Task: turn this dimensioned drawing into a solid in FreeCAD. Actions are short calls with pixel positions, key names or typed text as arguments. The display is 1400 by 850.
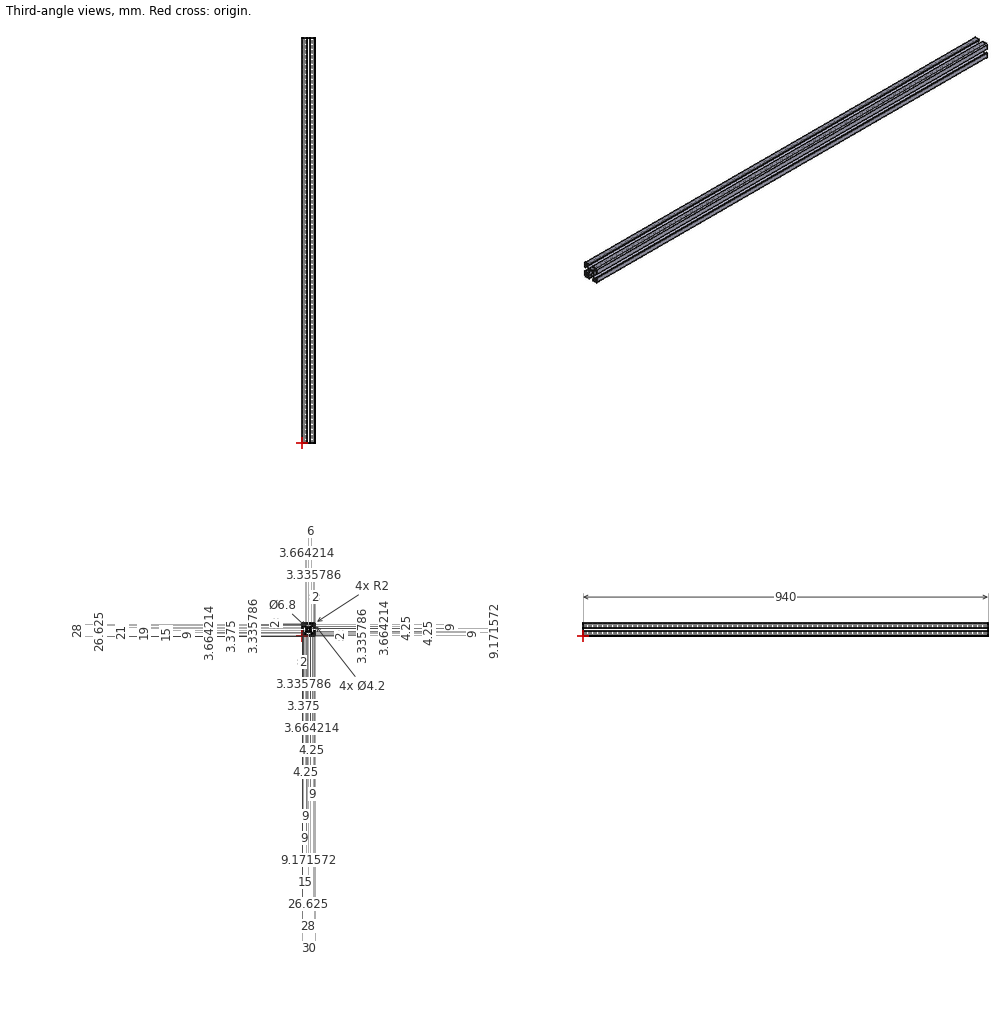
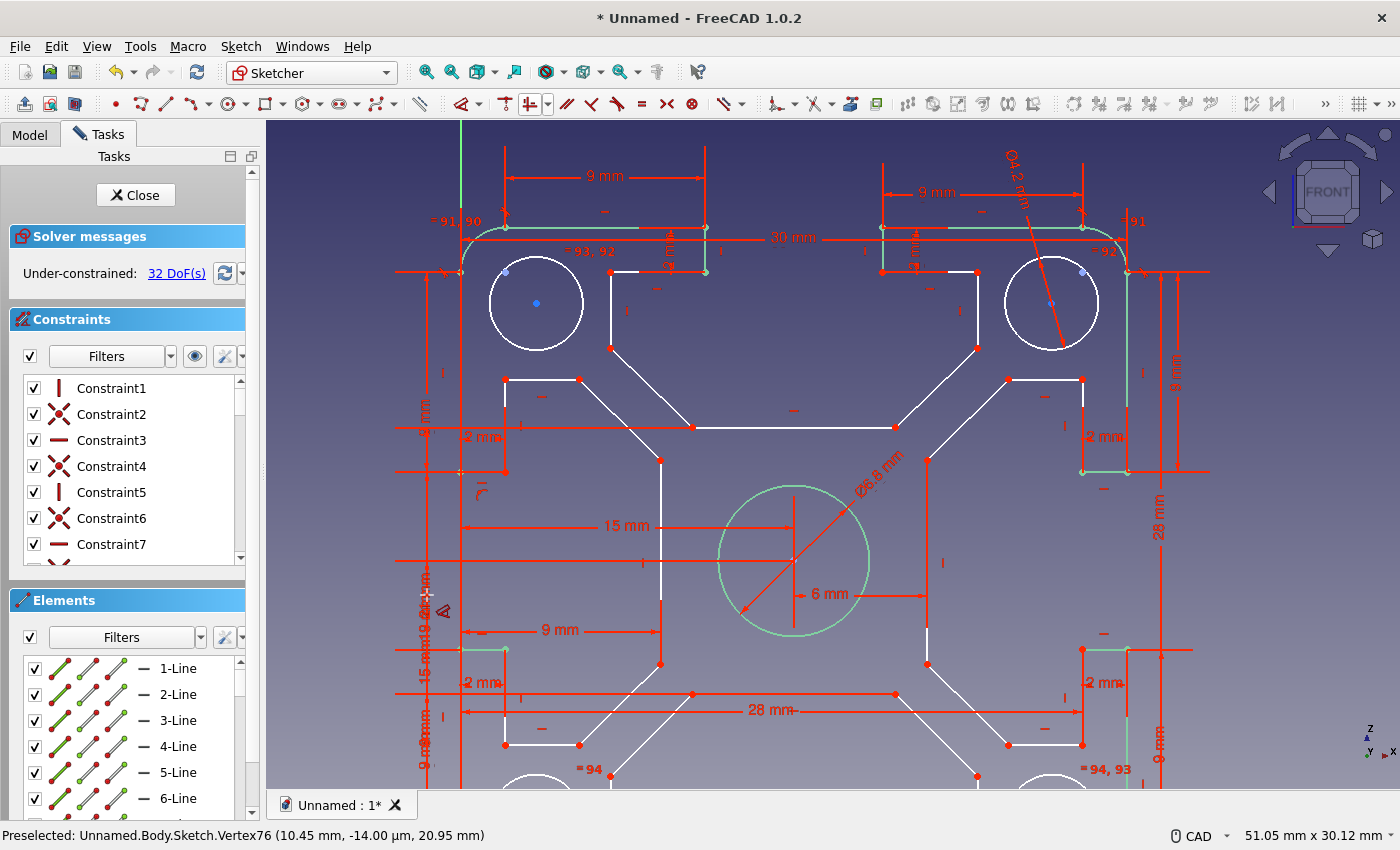
click(1083, 444)
click(1049, 405)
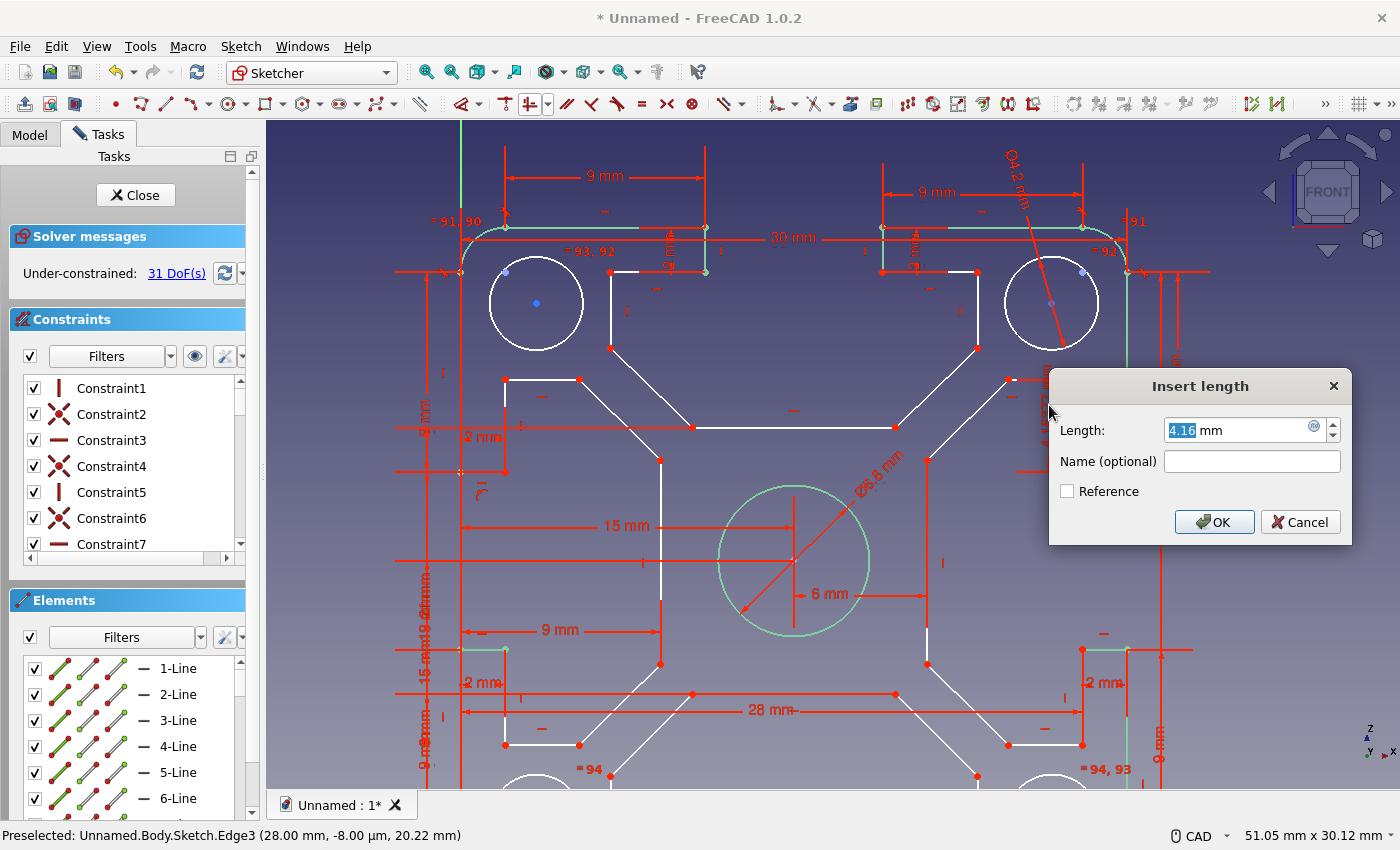
text(4.25)
key(Return)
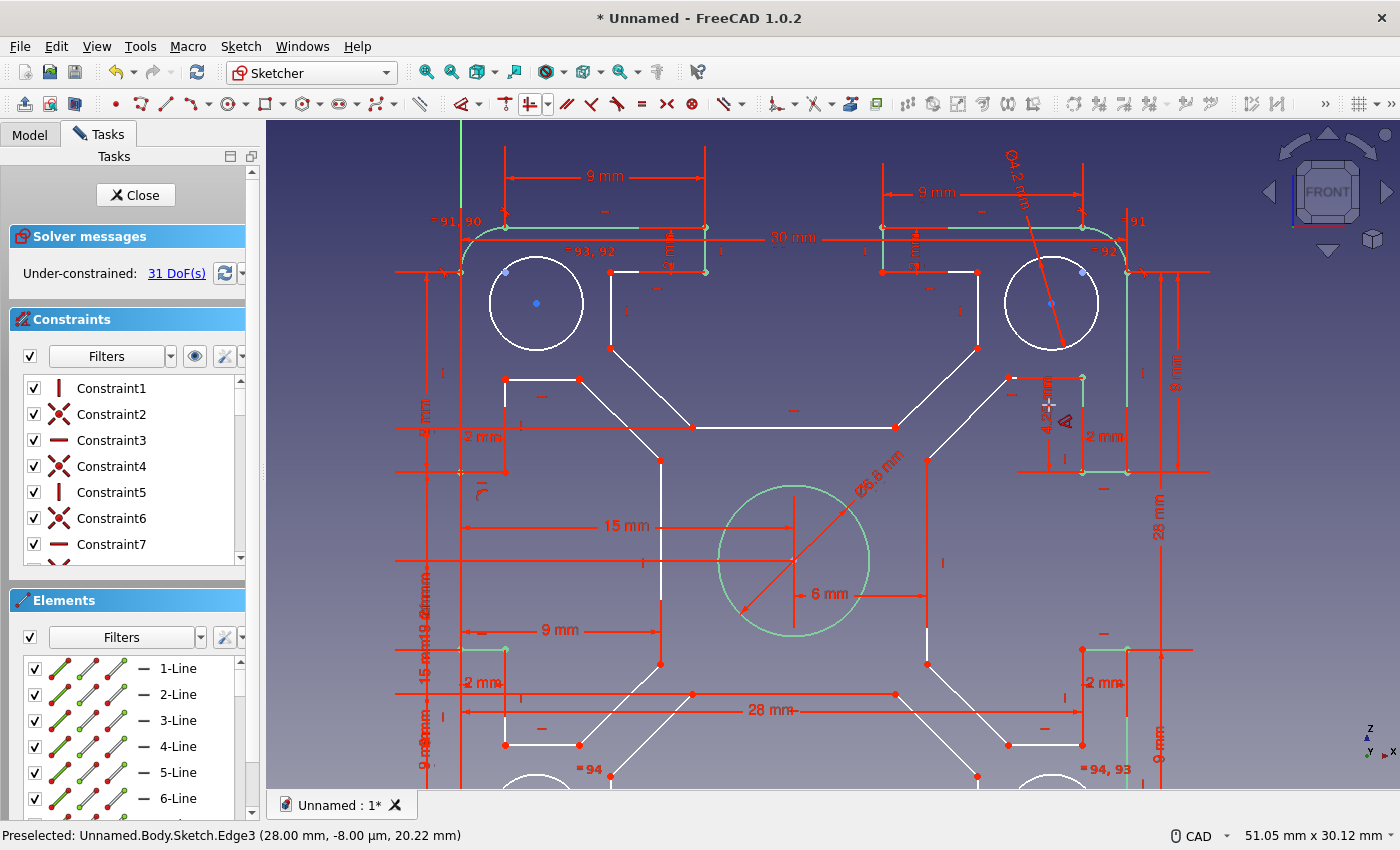
click(1083, 717)
click(1049, 719)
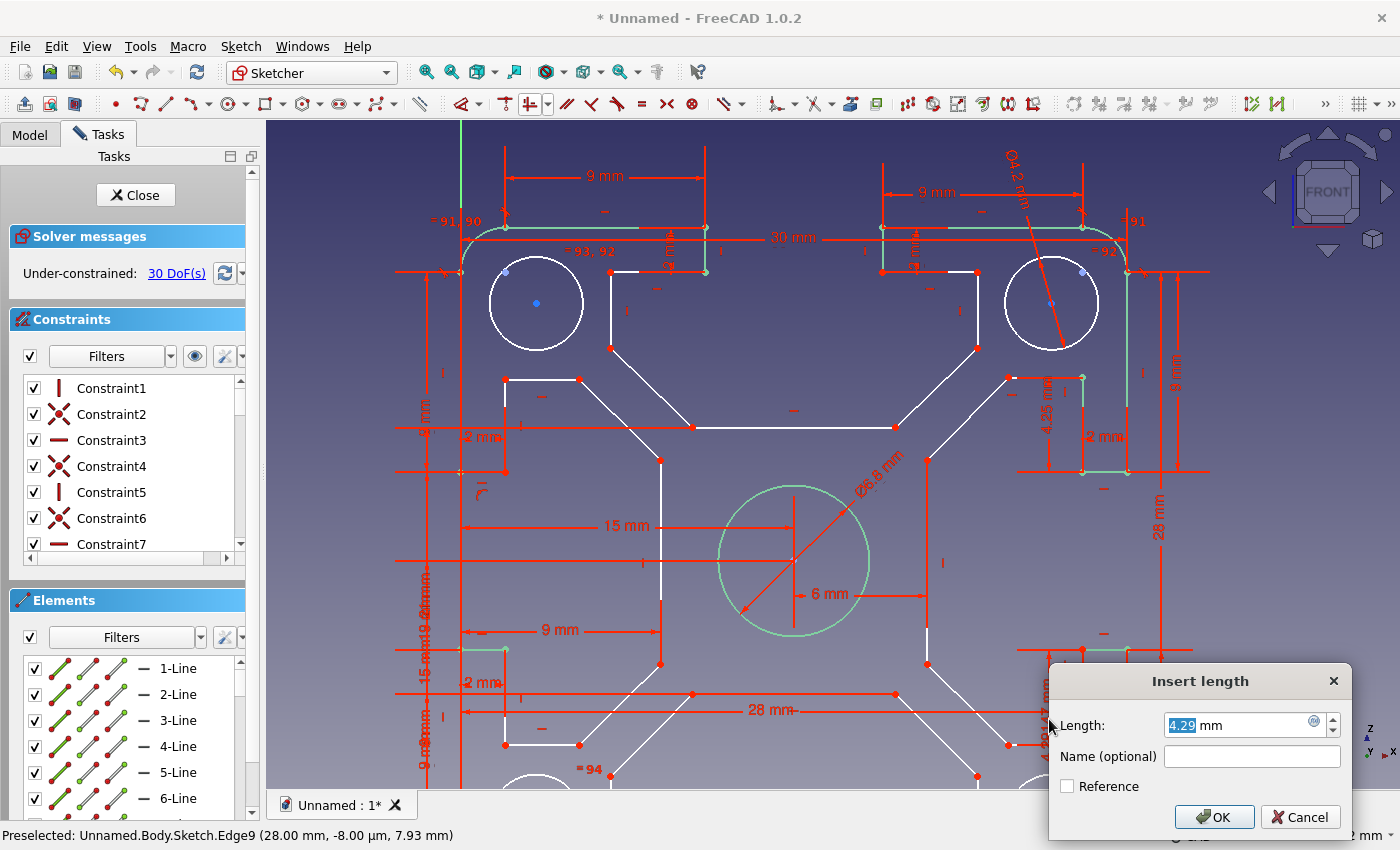
text(4.25)
key(Return)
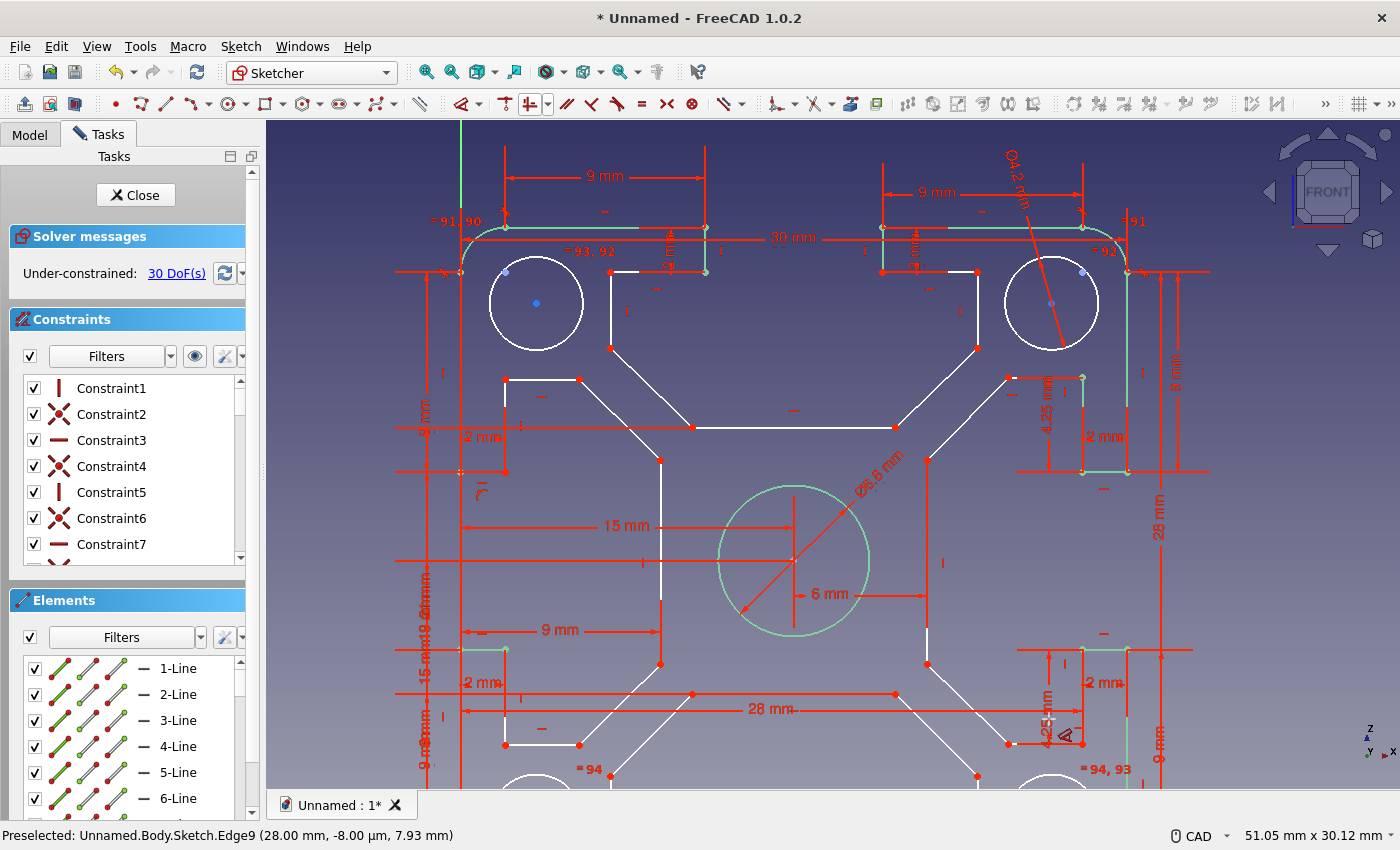
scroll(705, 238, down, 2)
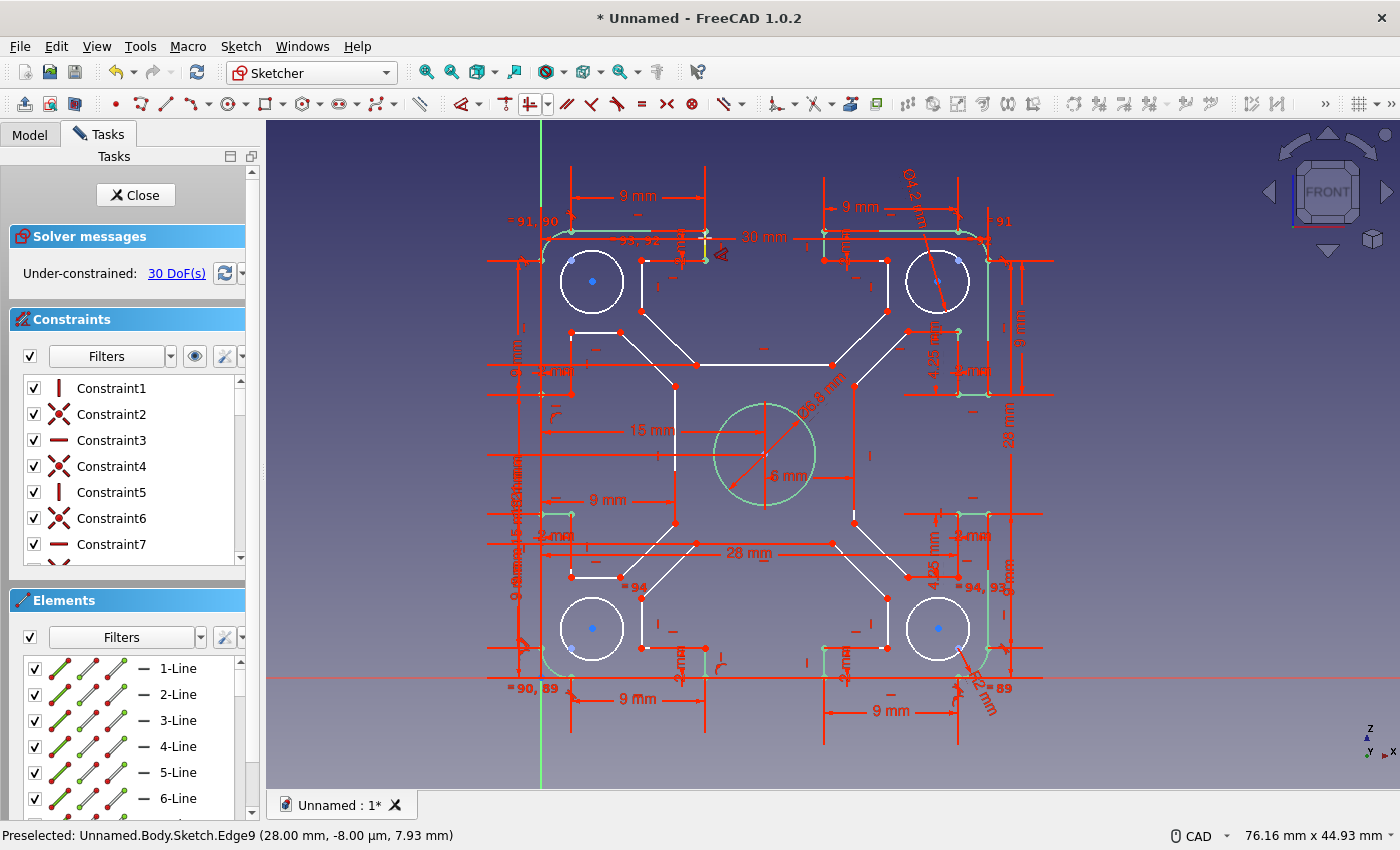
click(843, 648)
click(856, 614)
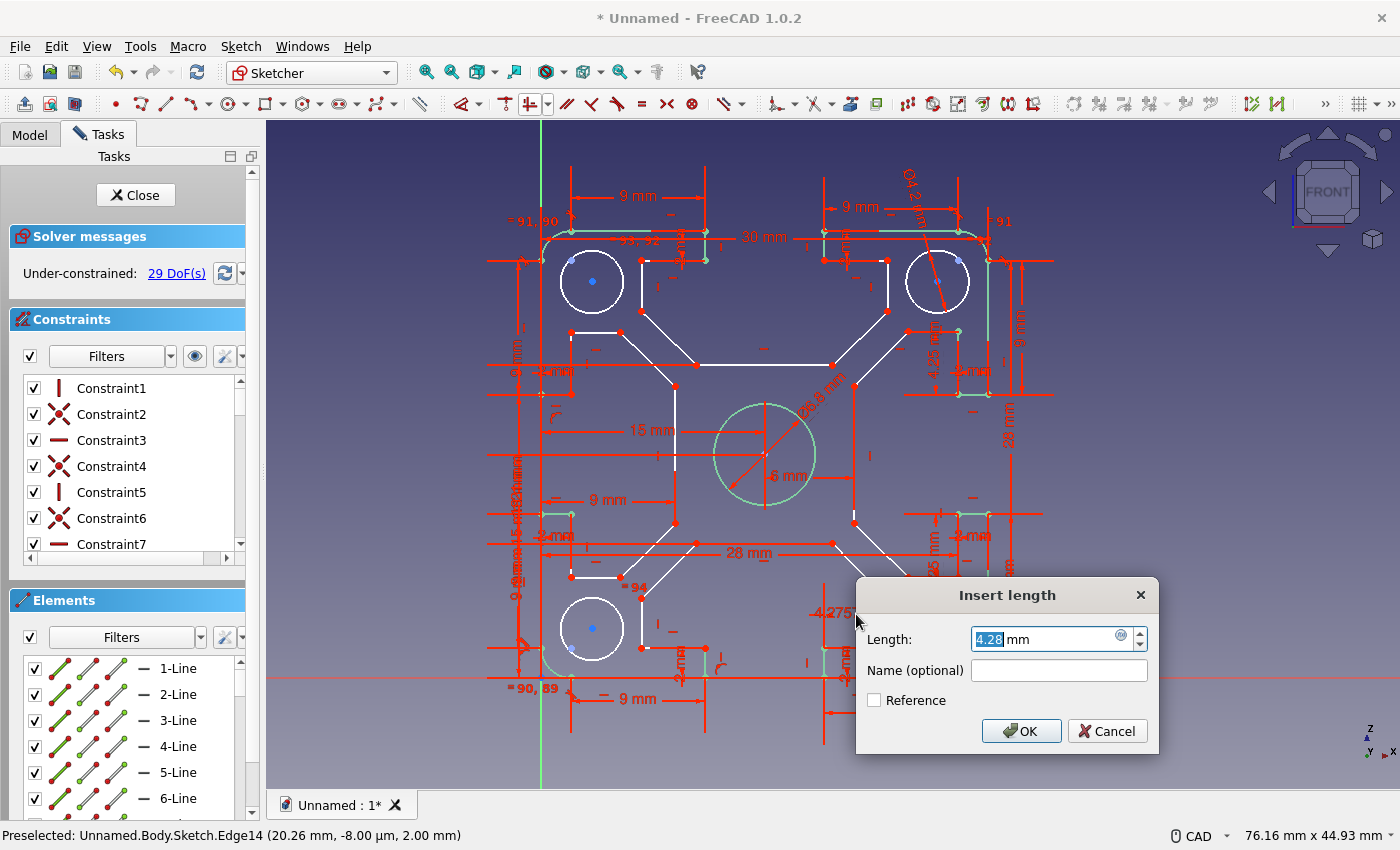
text(4.25)
key(Return)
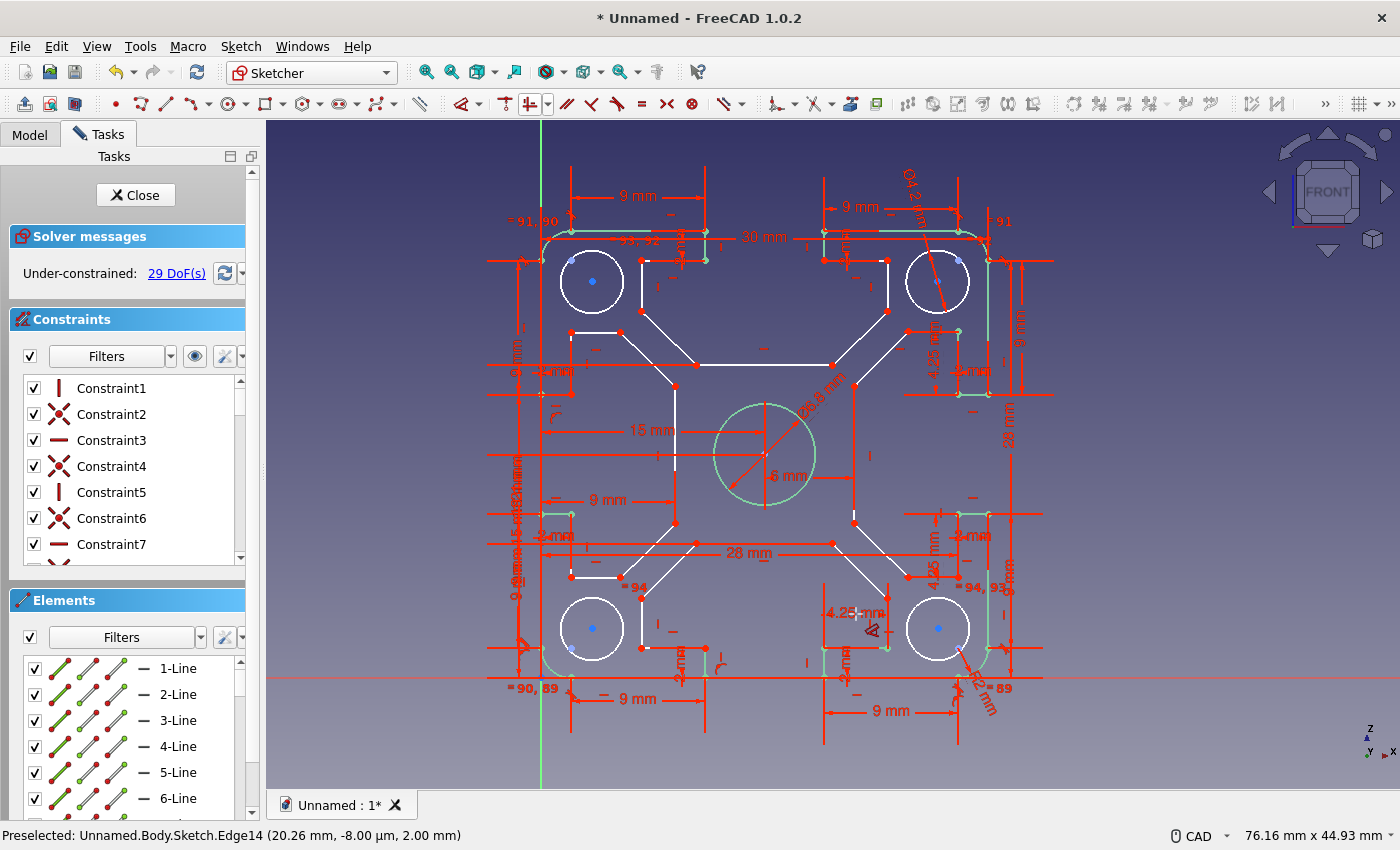
click(661, 648)
click(674, 614)